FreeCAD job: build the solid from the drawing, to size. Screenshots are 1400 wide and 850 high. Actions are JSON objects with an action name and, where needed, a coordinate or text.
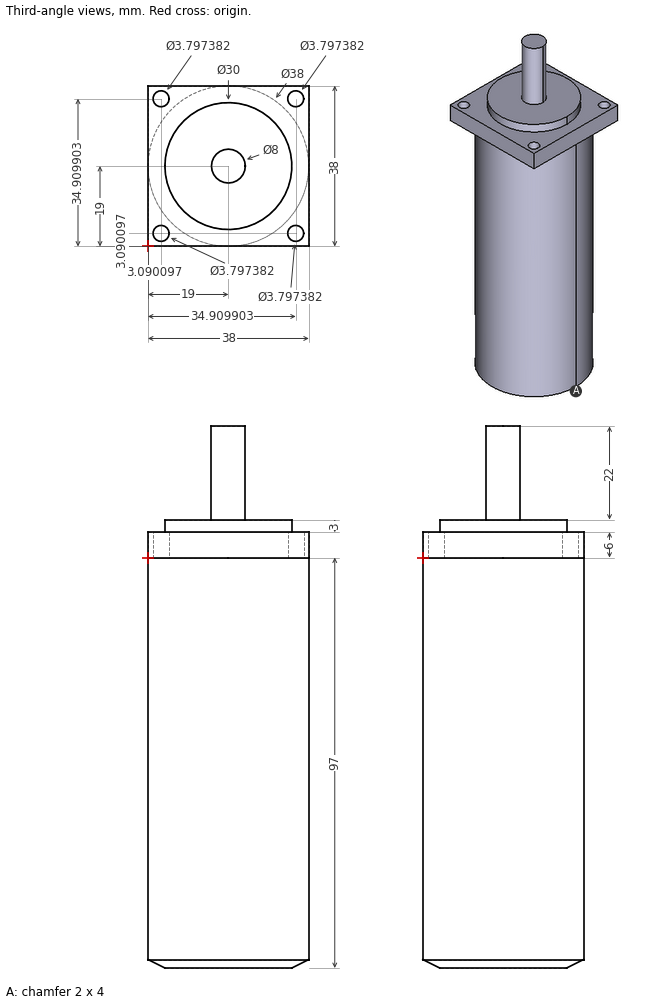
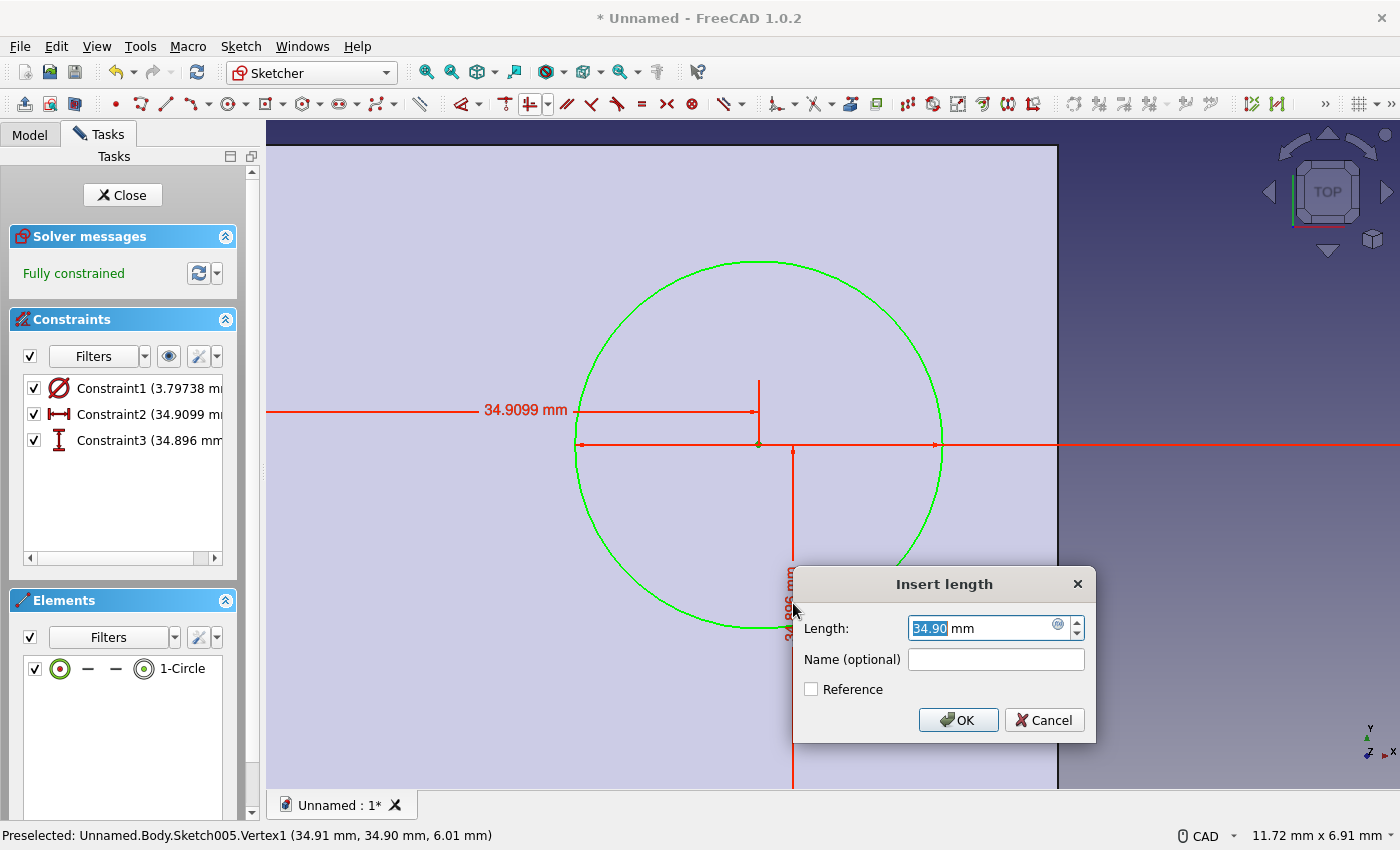
{"action": "type", "text": "34.909903"}
{"action": "key", "text": "Return"}
{"action": "key", "text": "Escape"}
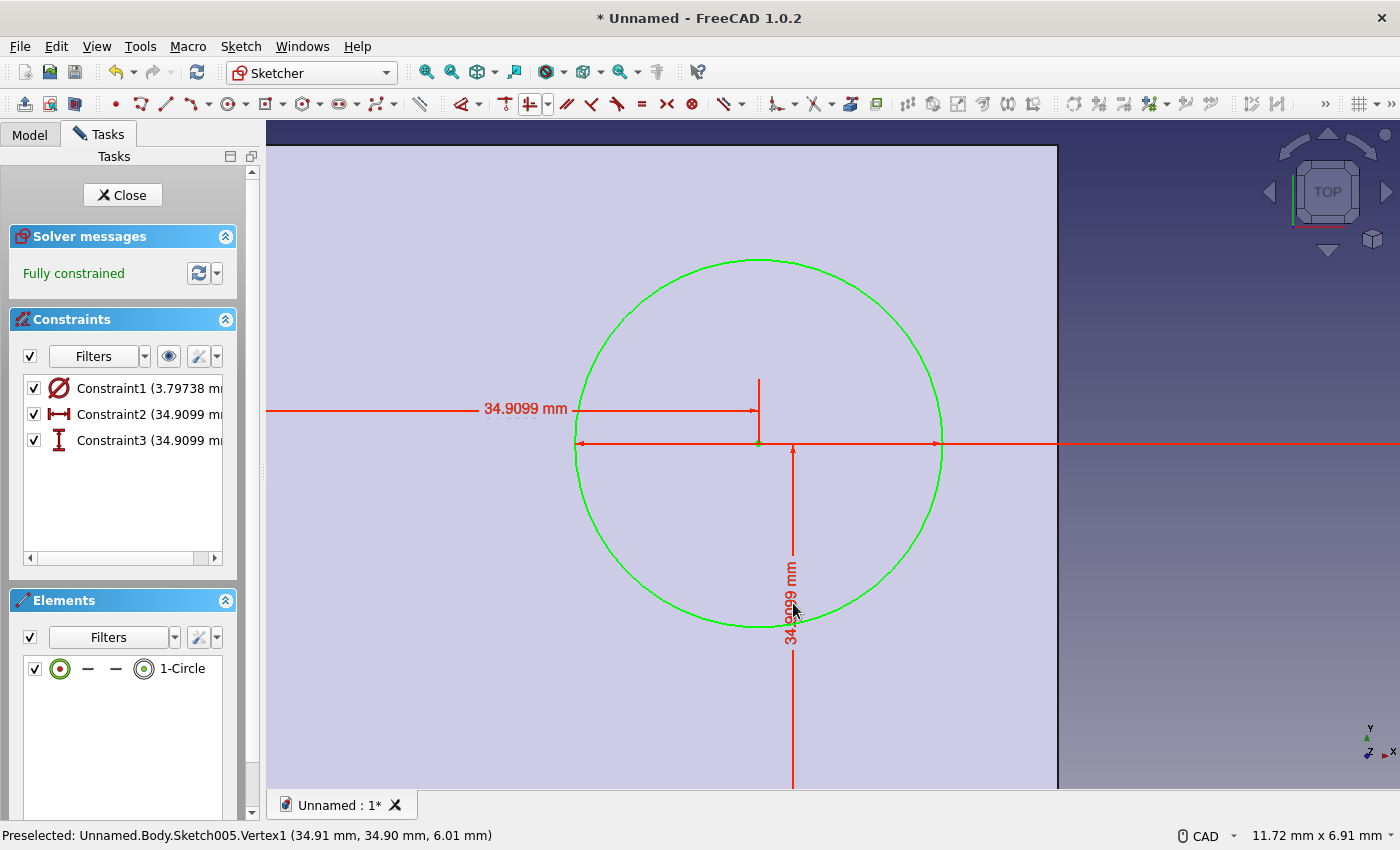
{"action": "left_click", "coordinate": [123, 195]}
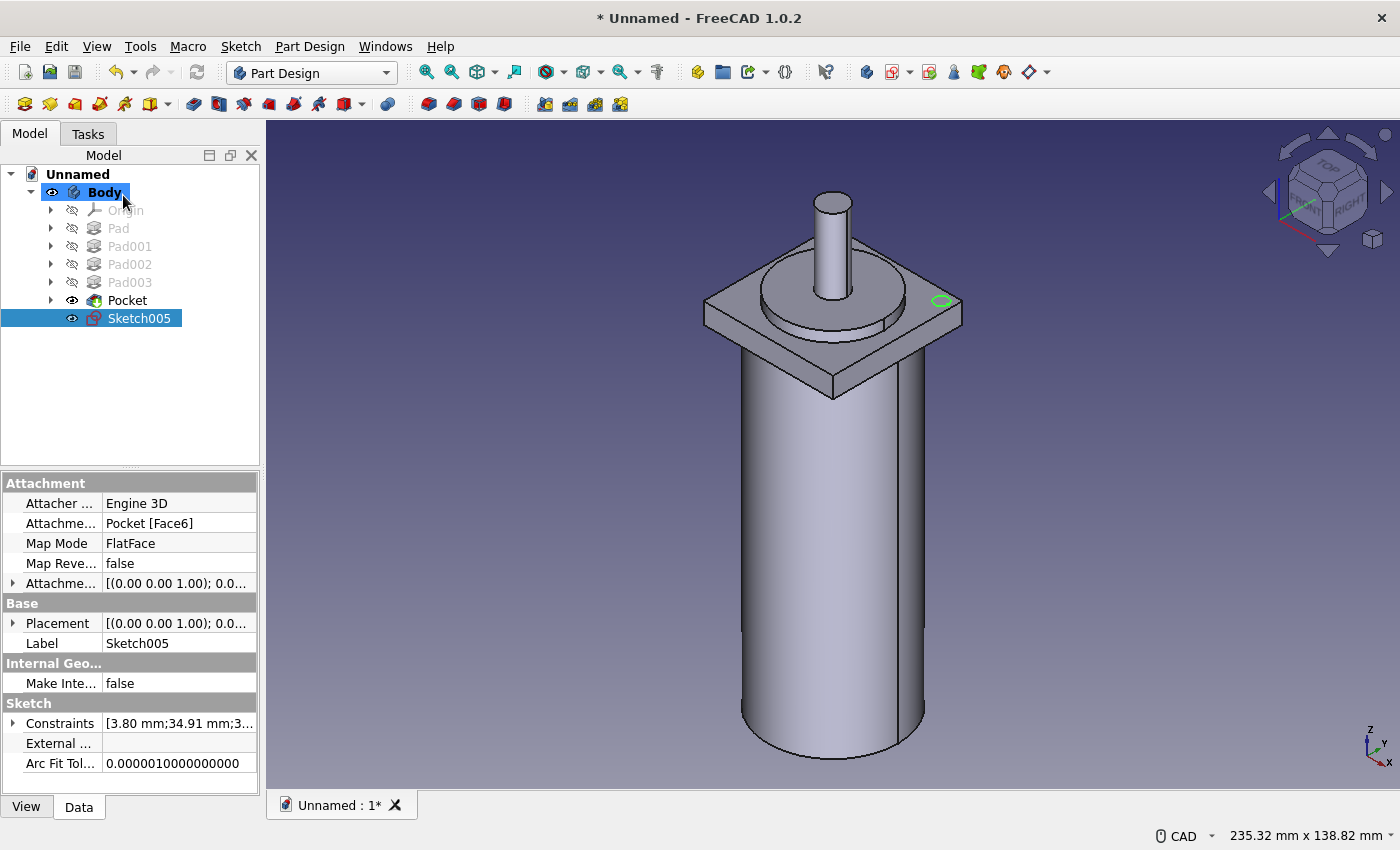
{"action": "left_click", "coordinate": [194, 104]}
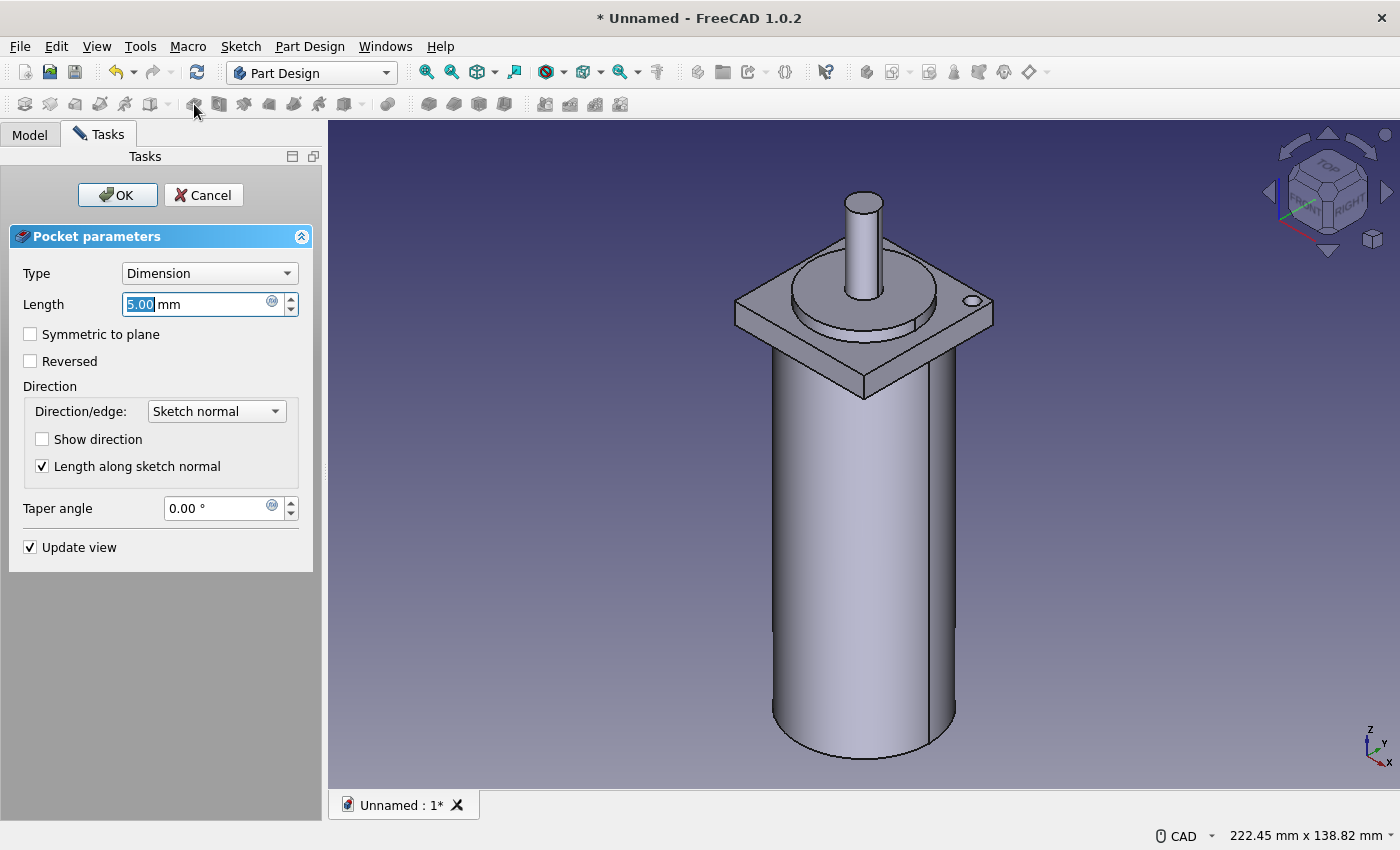
{"action": "left_click", "coordinate": [210, 274]}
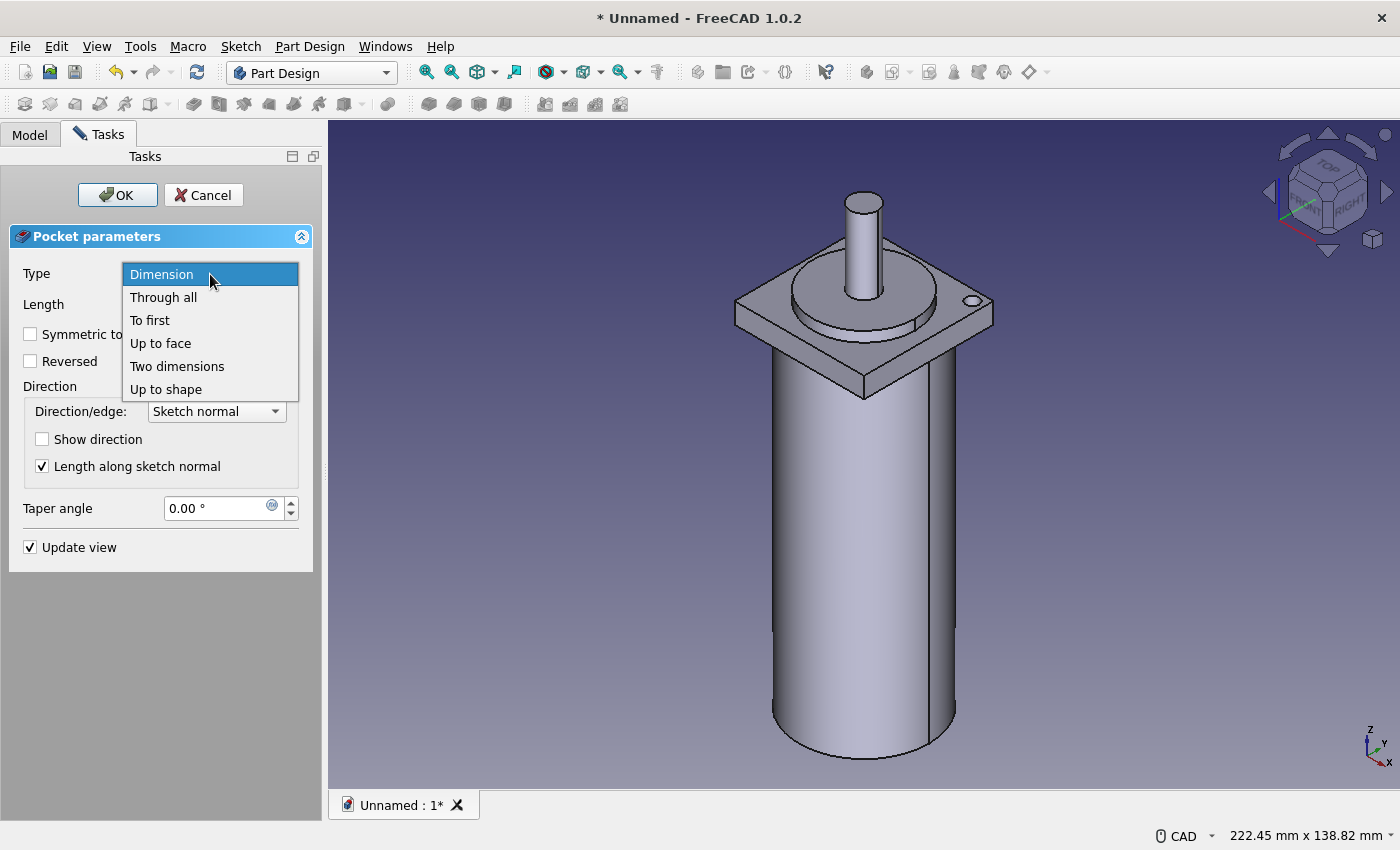
{"action": "left_click", "coordinate": [208, 320]}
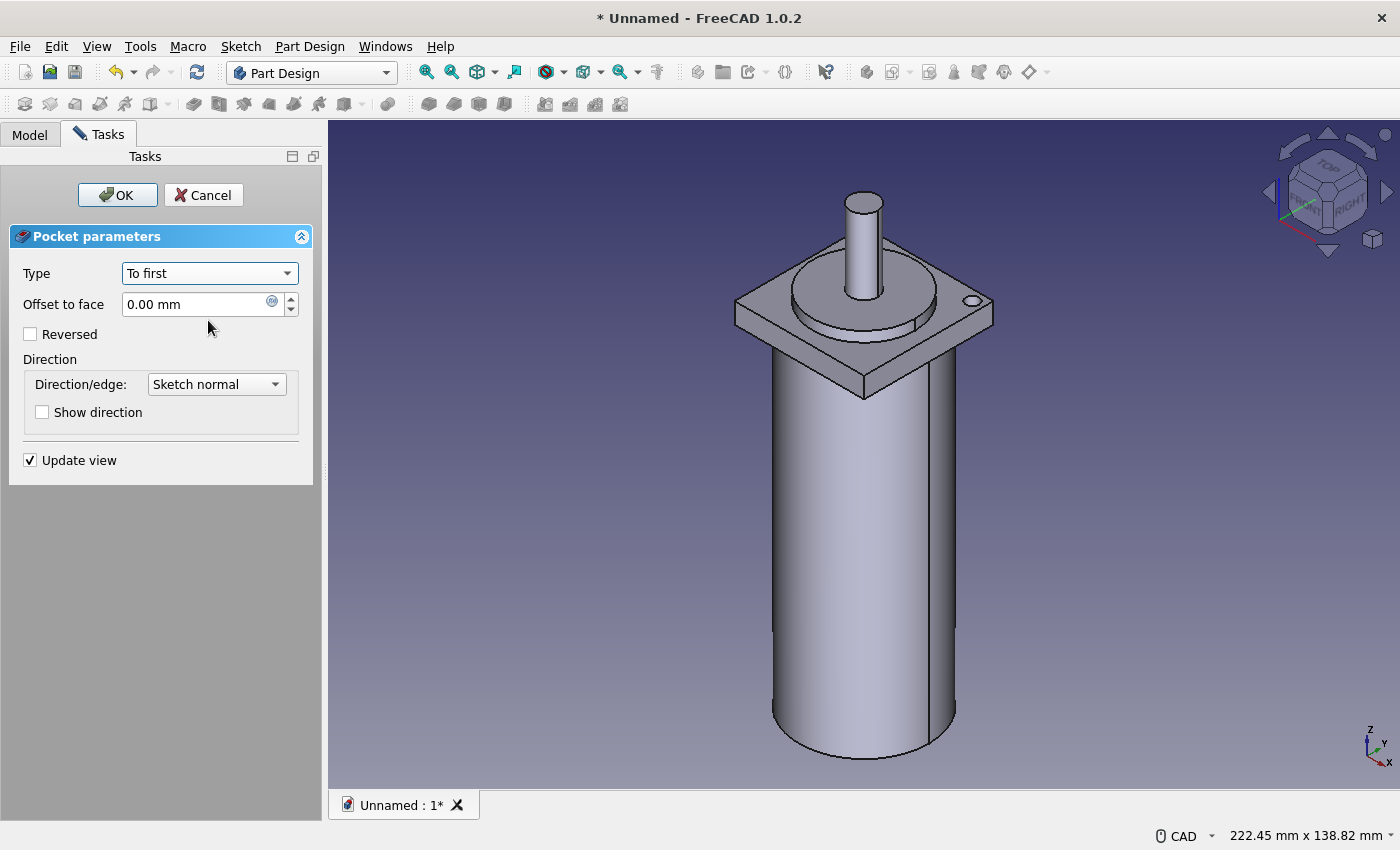
{"action": "left_click", "coordinate": [118, 195]}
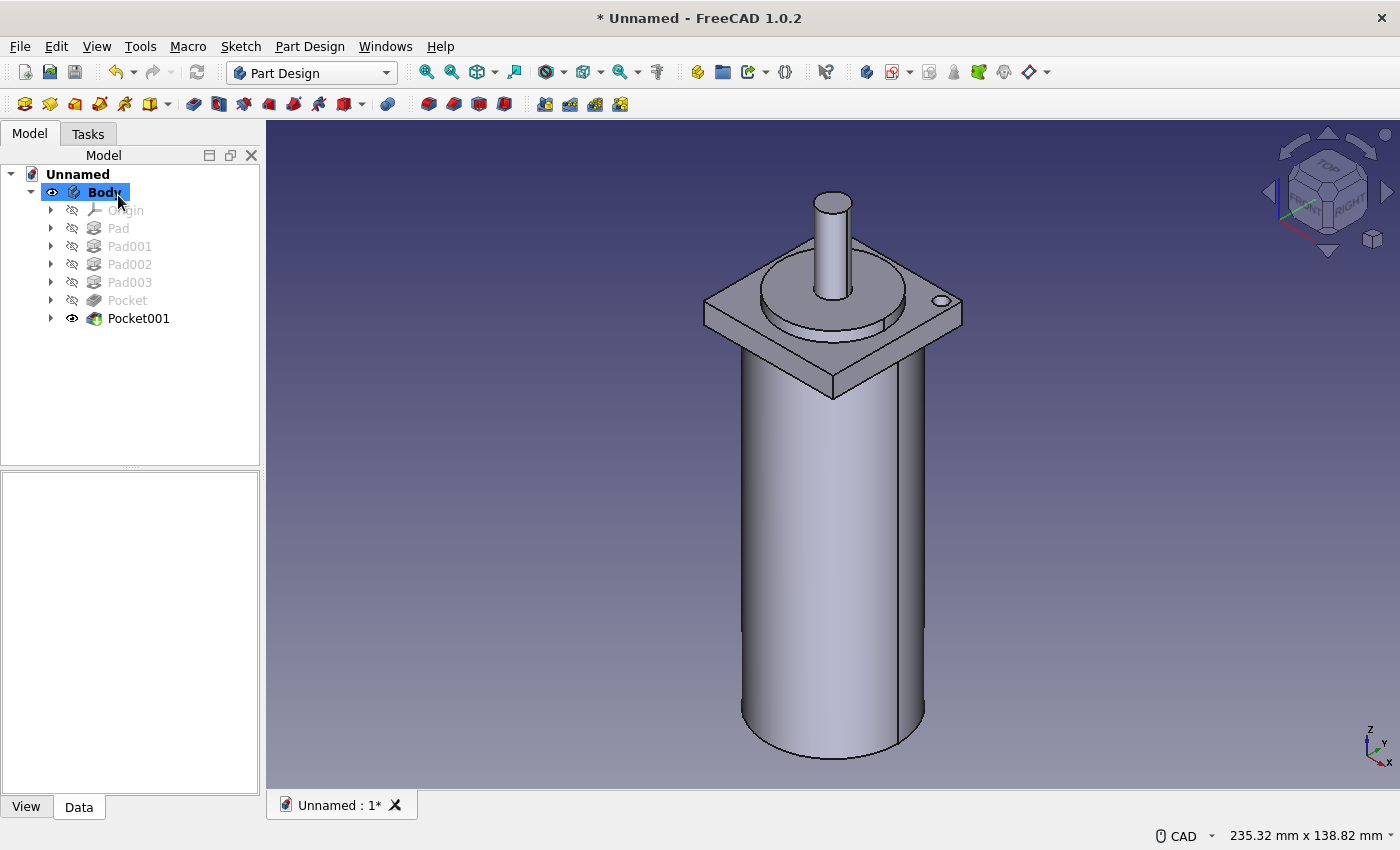
{"action": "left_click", "coordinate": [925, 311]}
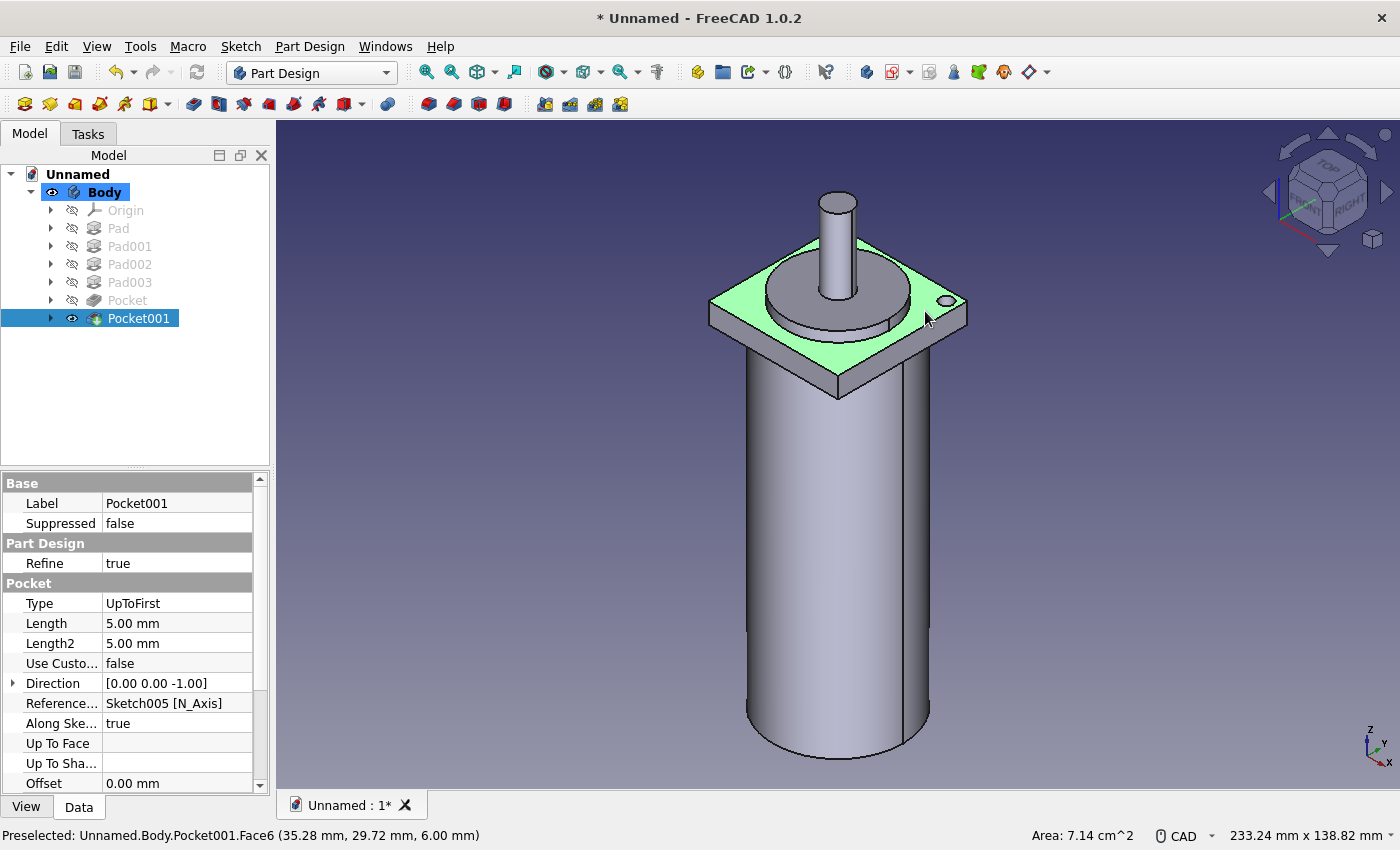
{"action": "left_click", "coordinate": [892, 72]}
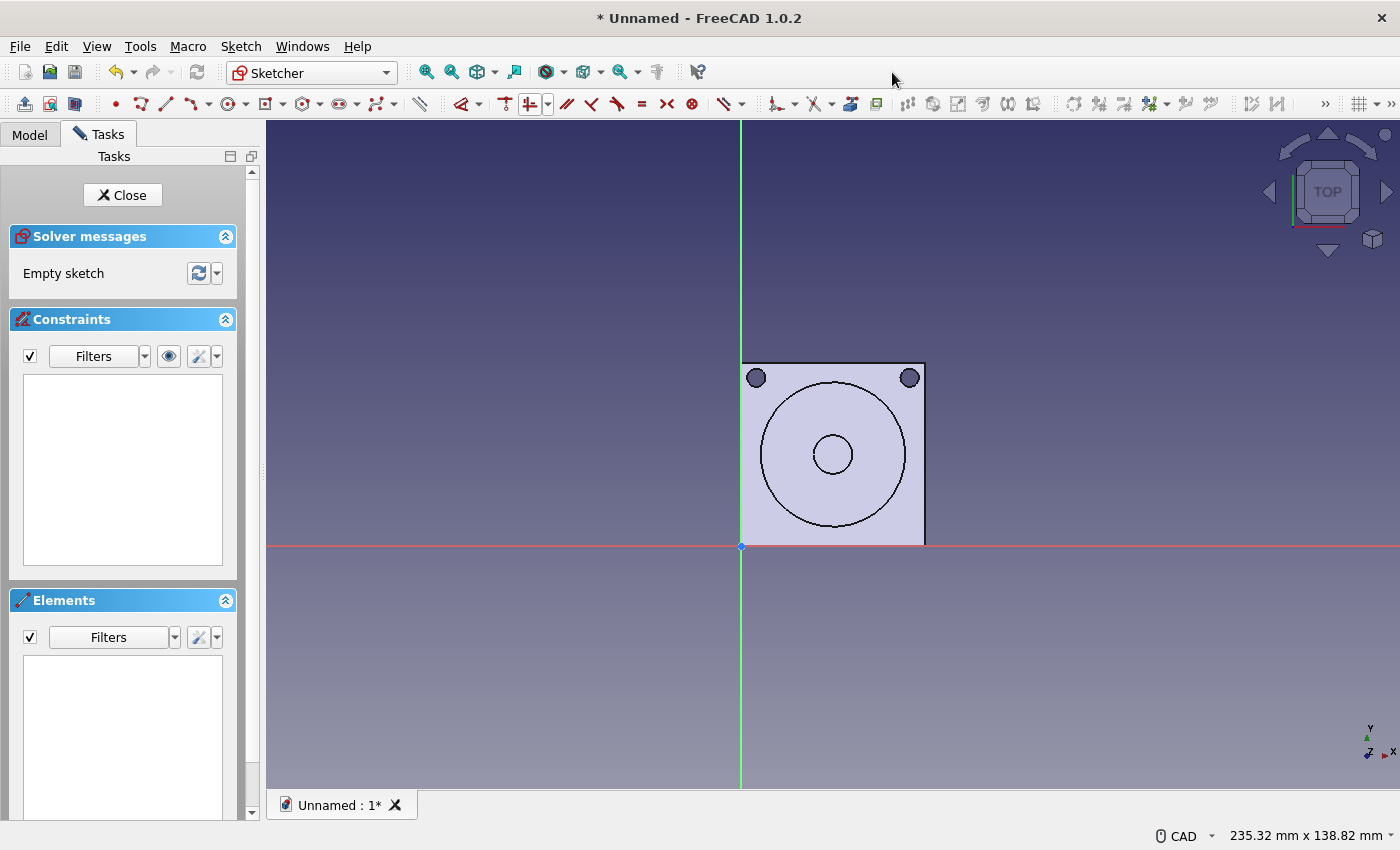
{"action": "scroll", "coordinate": [917, 535], "scroll_direction": "up", "scroll_amount": 15}